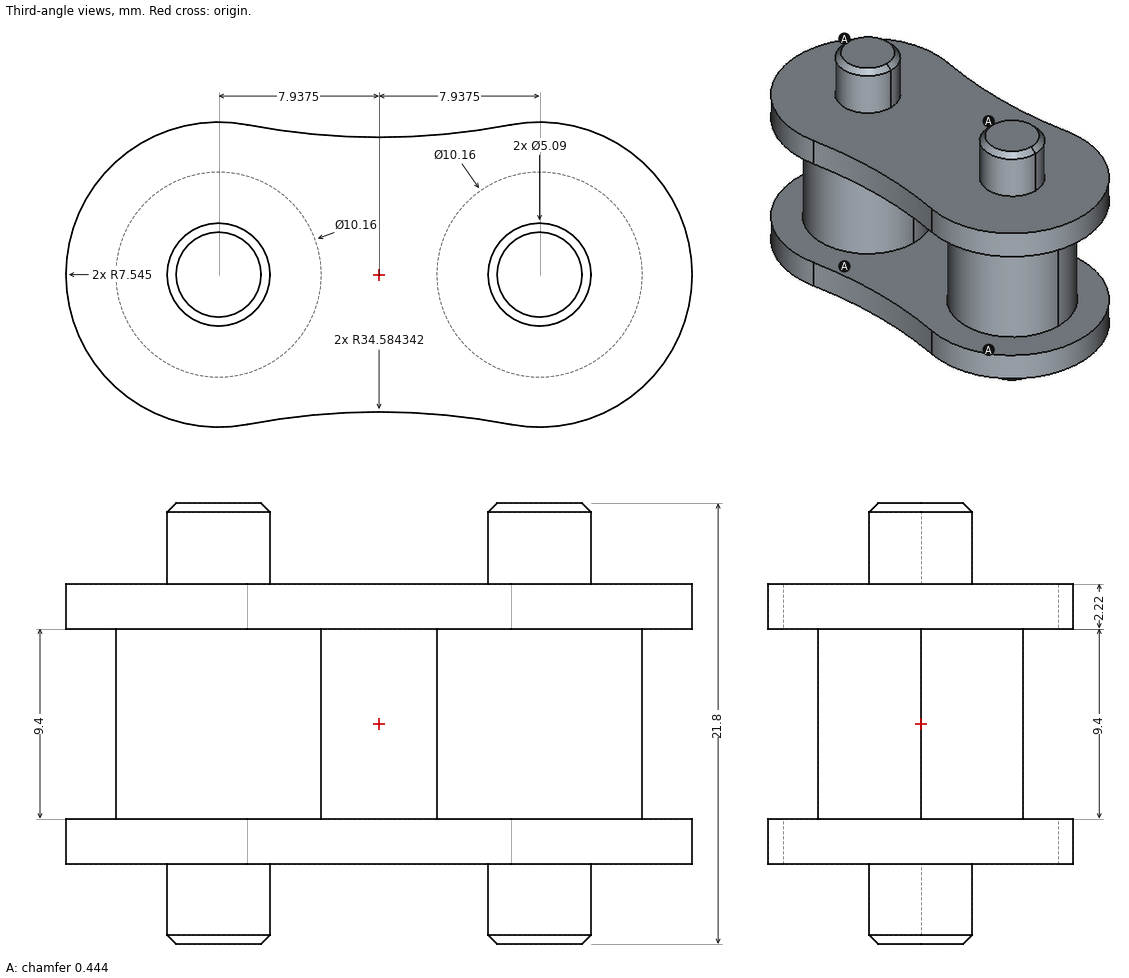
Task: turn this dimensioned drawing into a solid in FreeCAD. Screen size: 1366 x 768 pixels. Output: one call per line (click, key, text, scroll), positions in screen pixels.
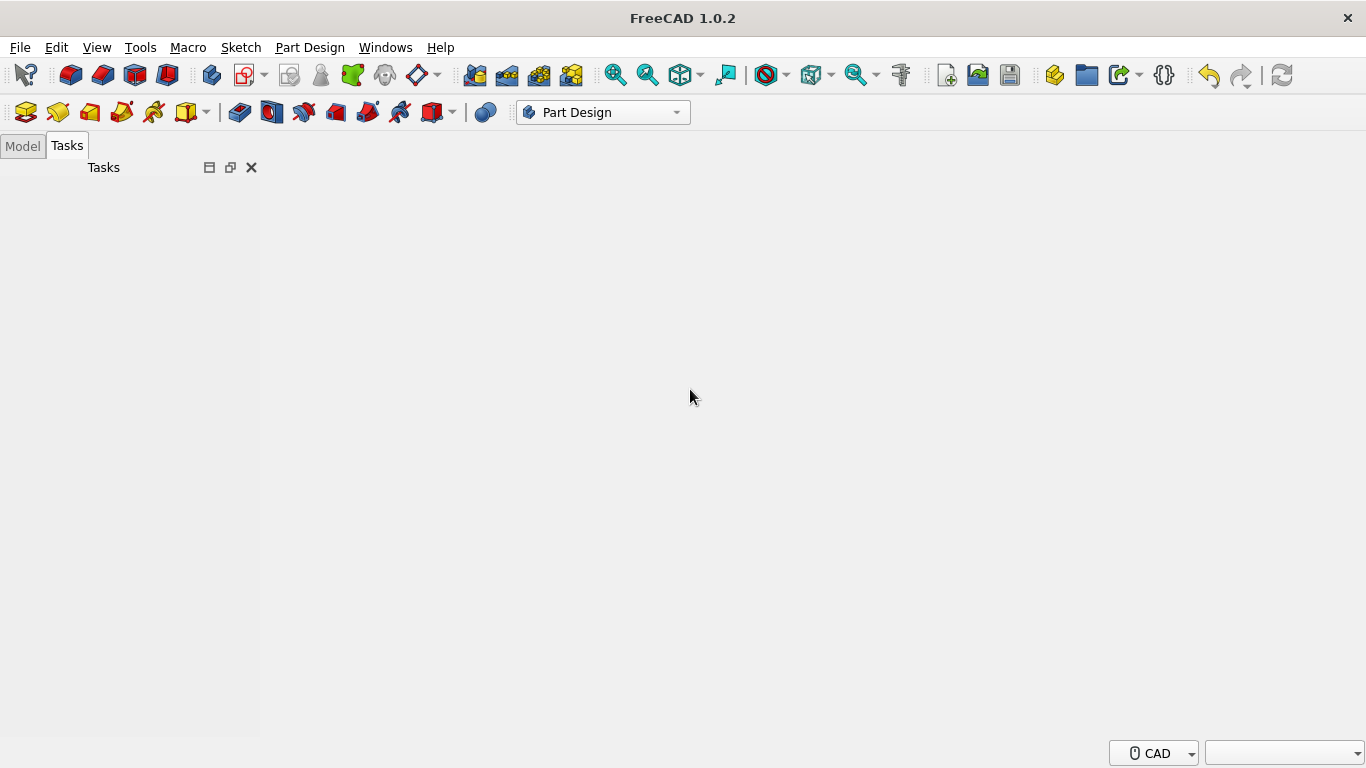
click(946, 76)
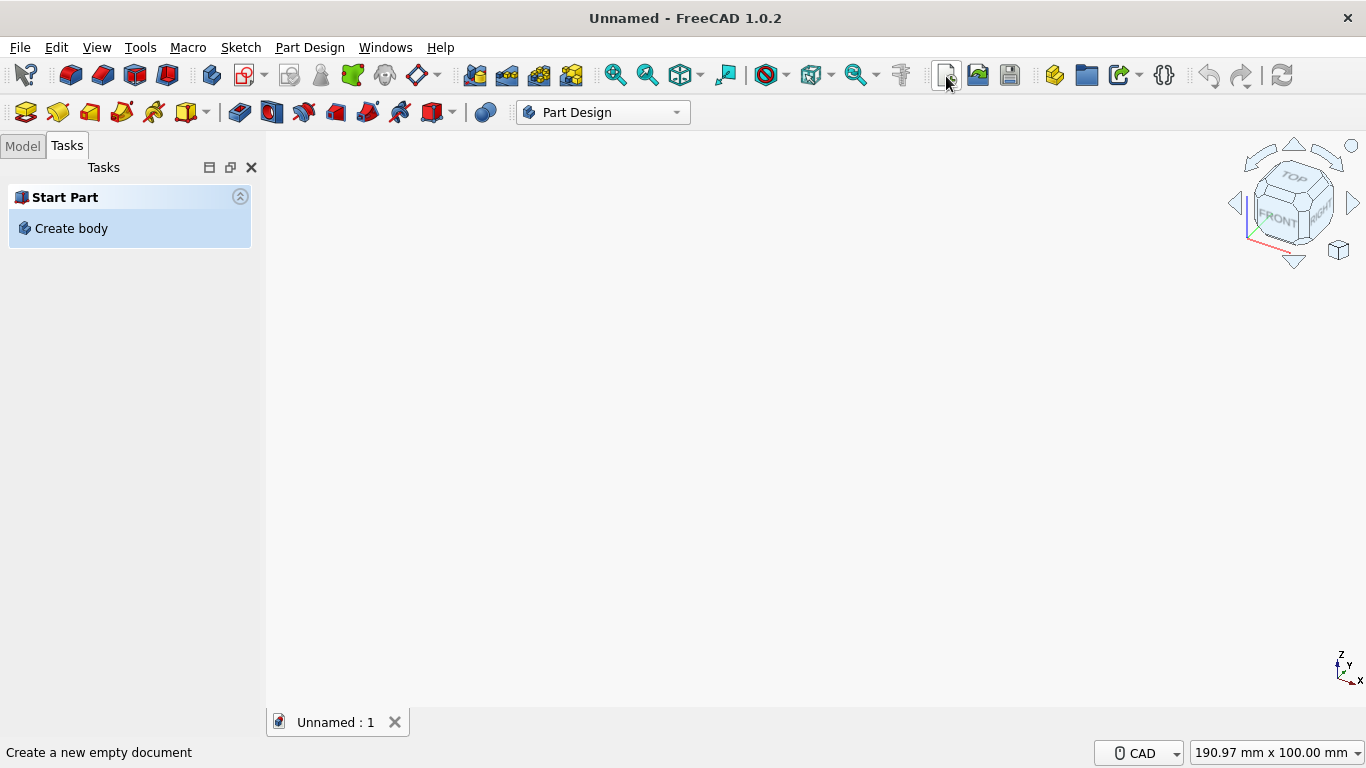
click(244, 76)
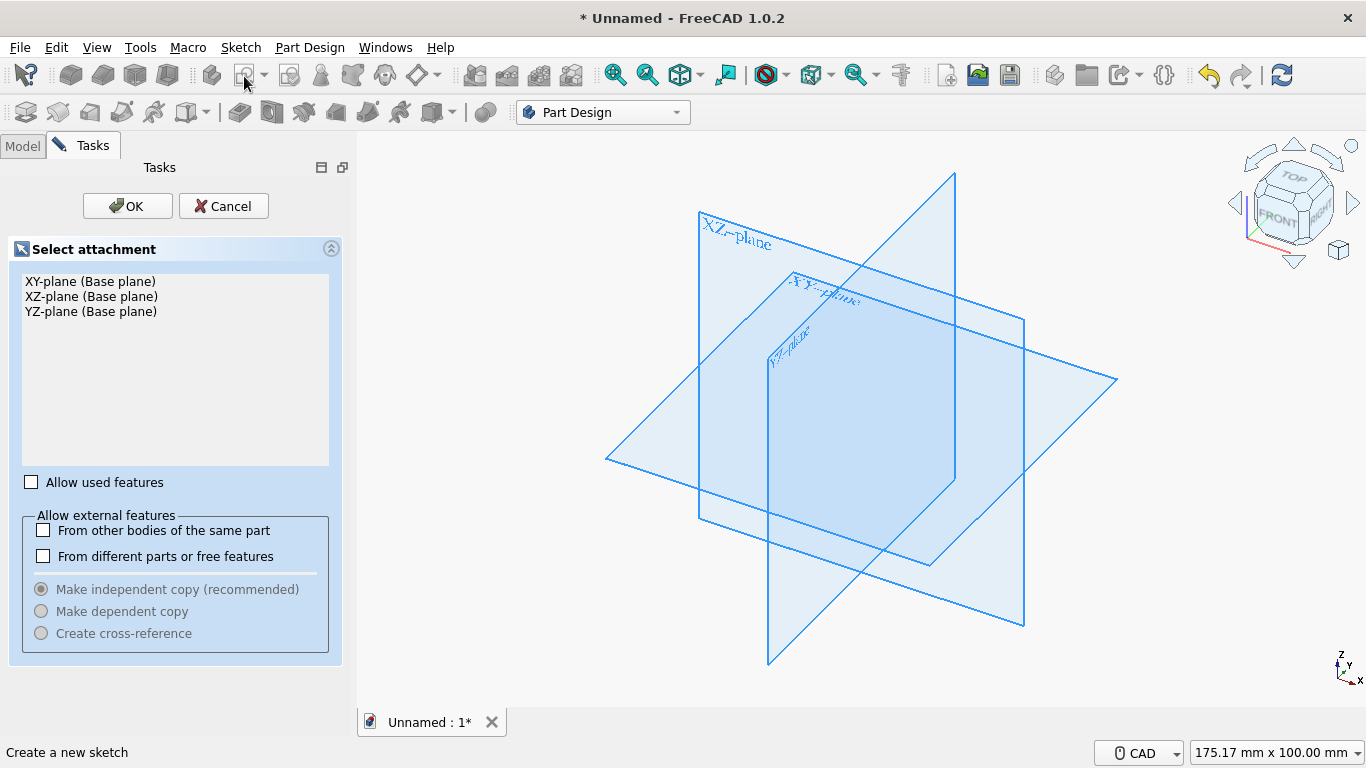
click(82, 282)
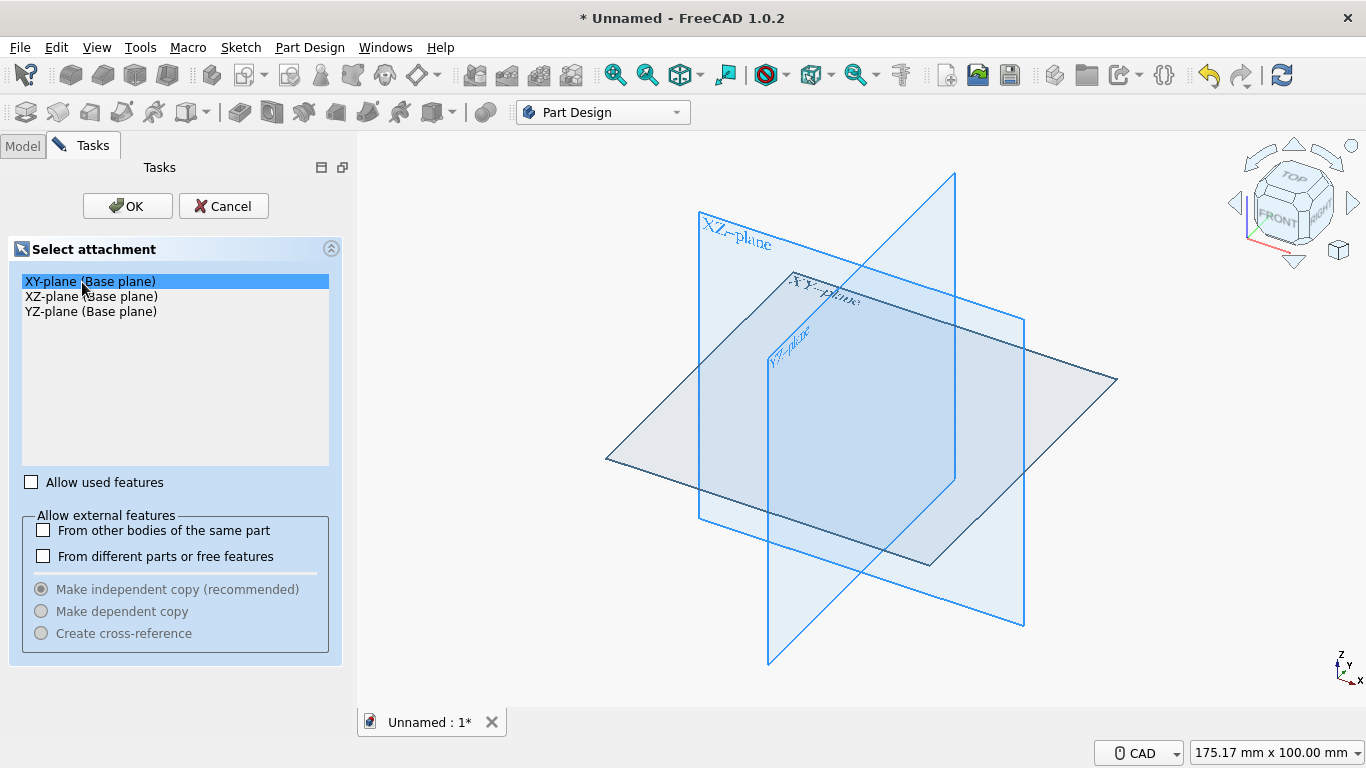
click(128, 206)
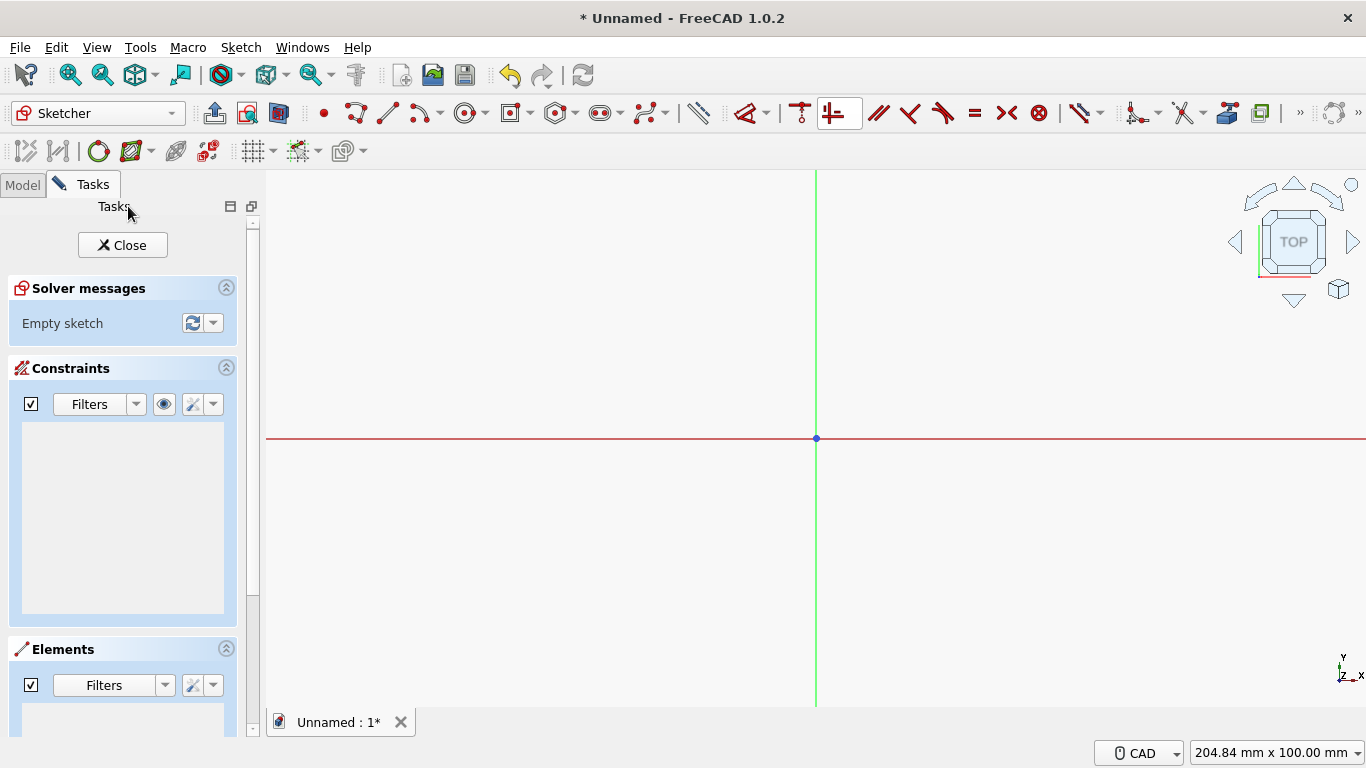
scroll(871, 438, up, 9)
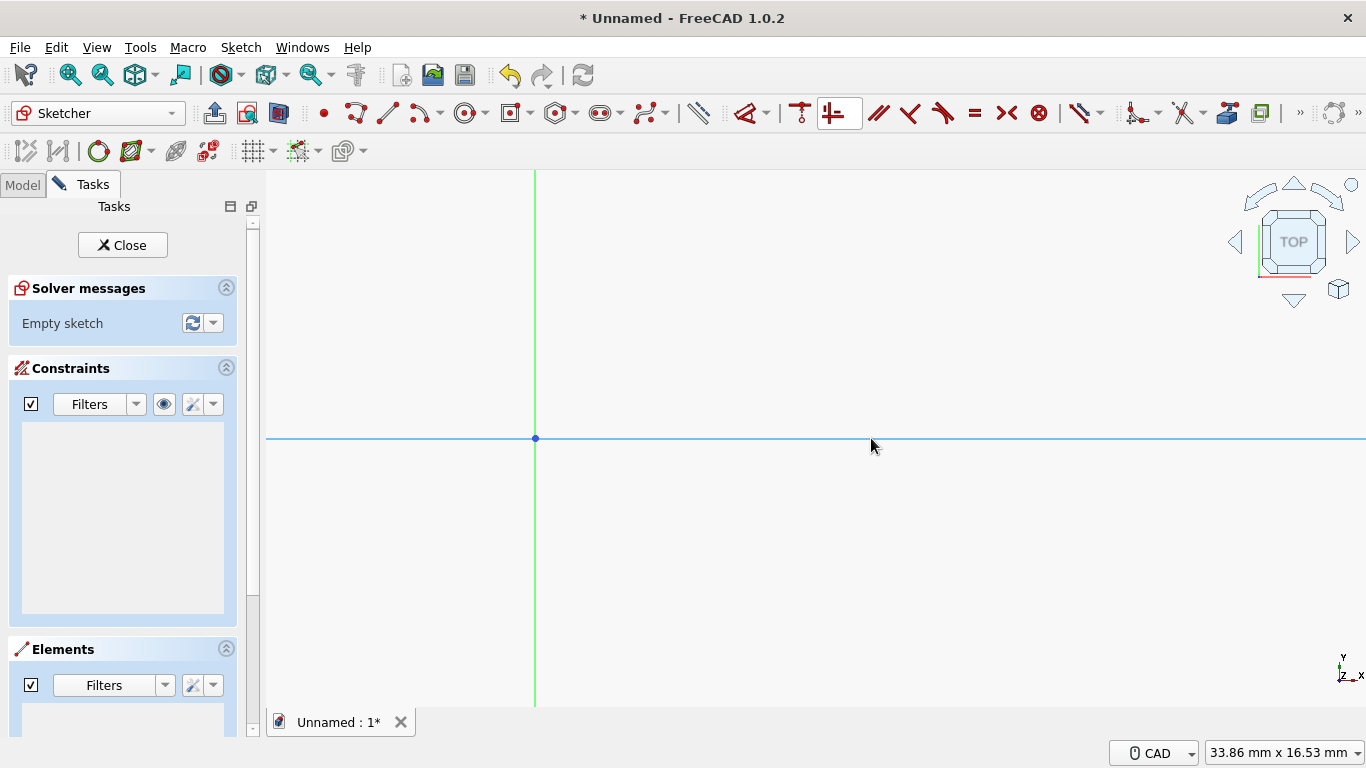
click(466, 114)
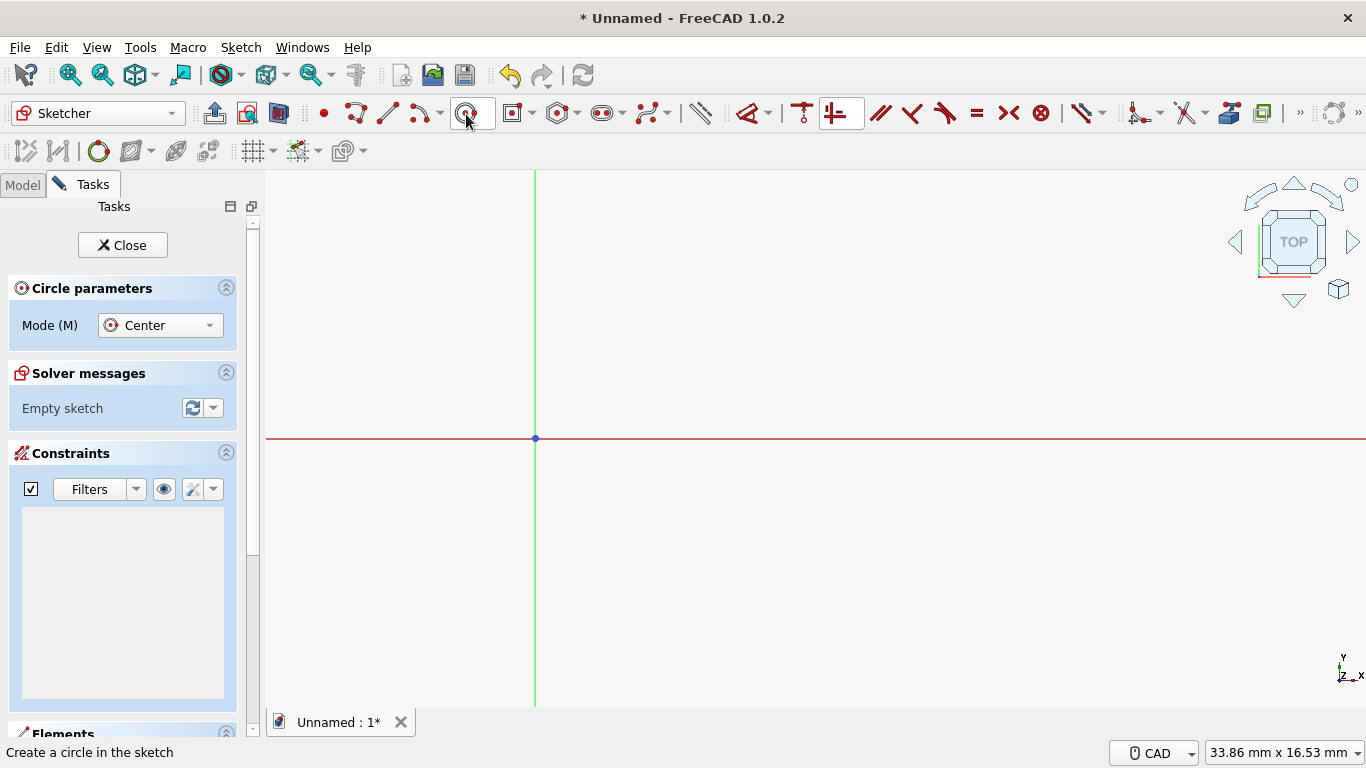
click(793, 438)
move(910, 322)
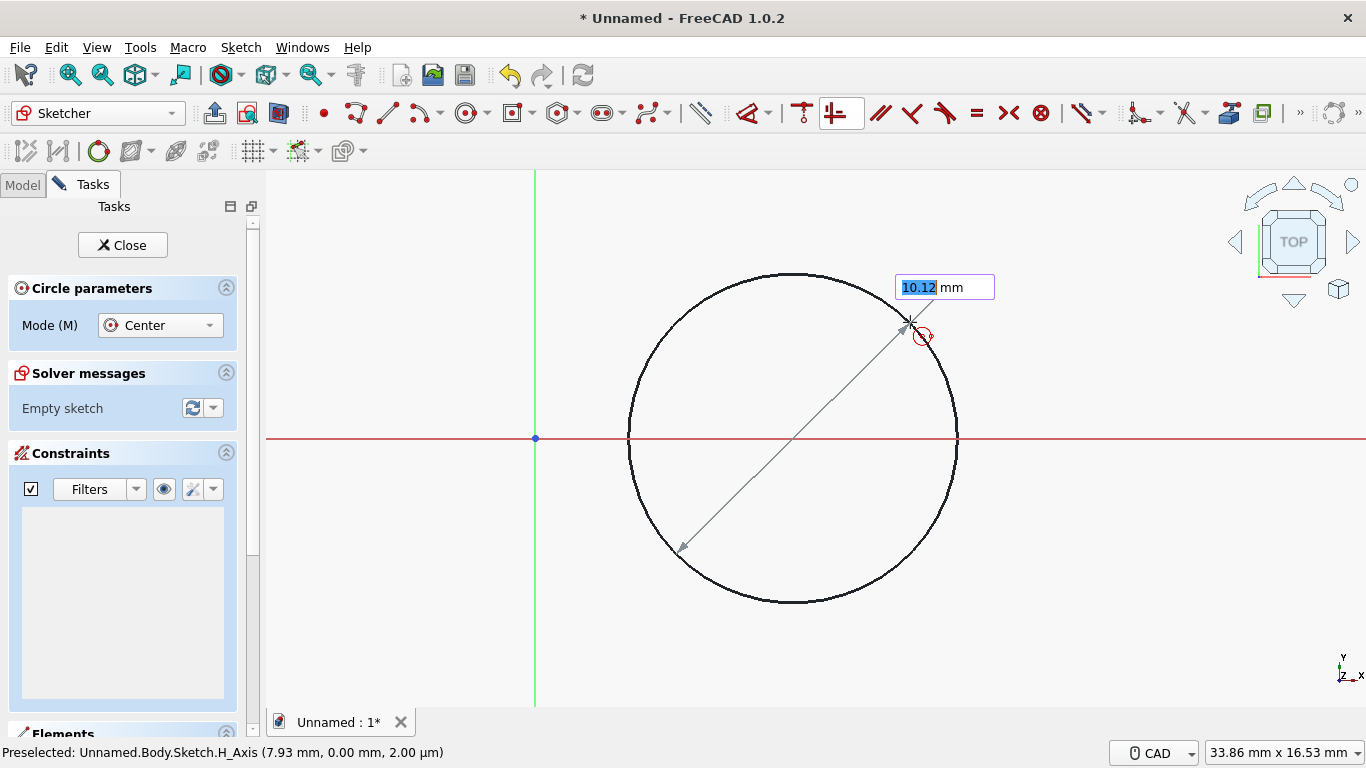
text(10.16)
key(Return)
key(Escape)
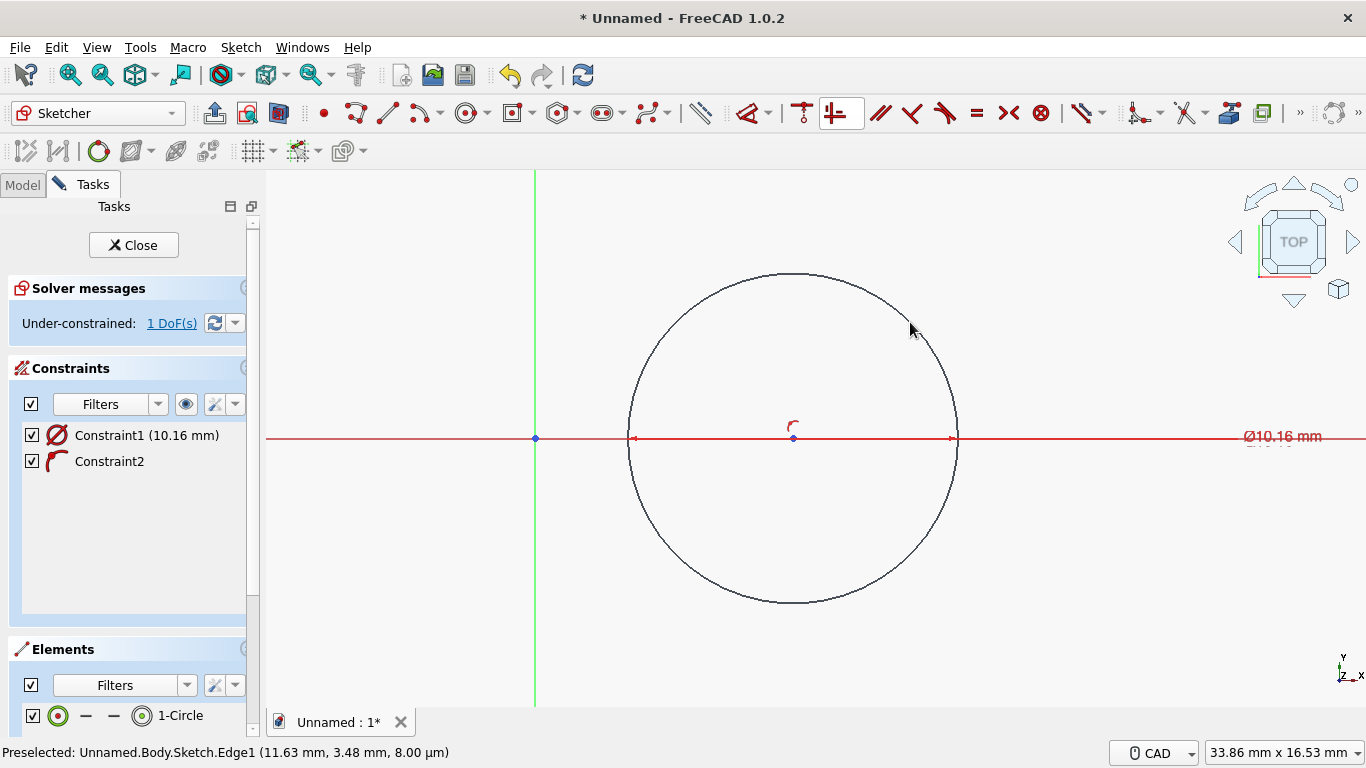
key(d)